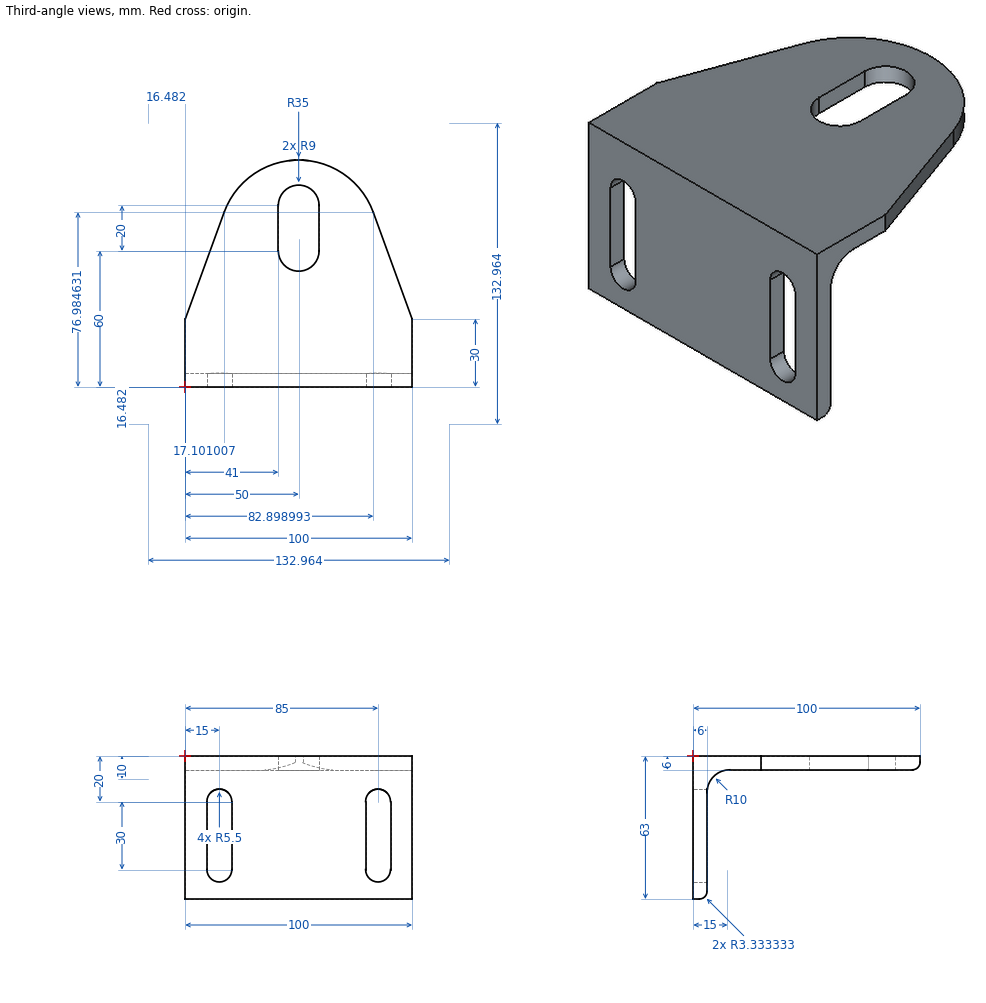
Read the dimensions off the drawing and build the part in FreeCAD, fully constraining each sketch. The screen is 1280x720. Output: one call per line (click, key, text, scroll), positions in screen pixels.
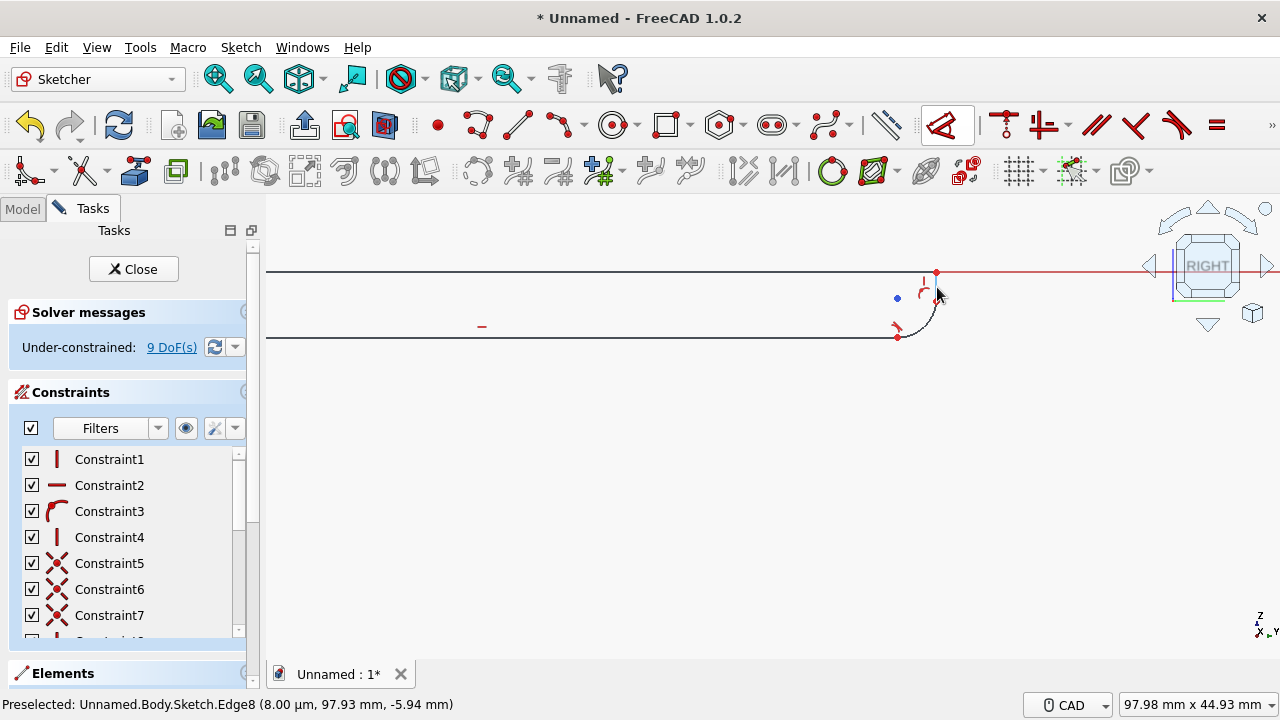
click(936, 287)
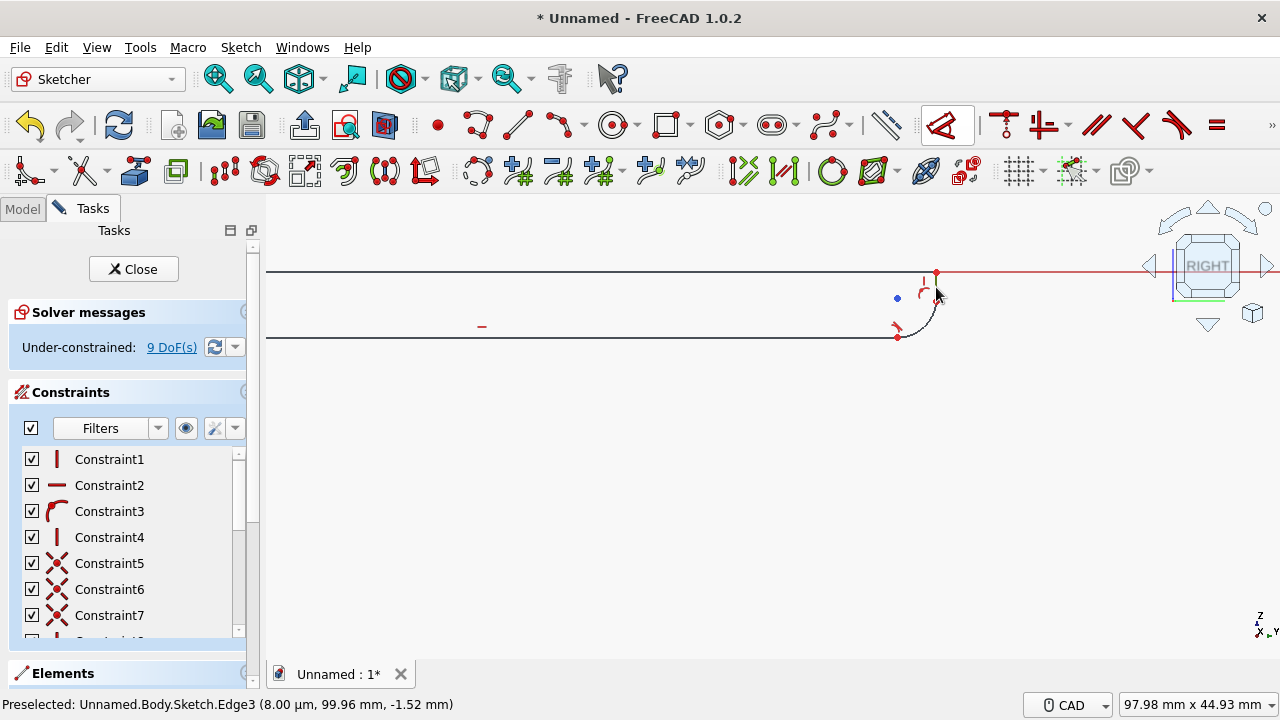
click(914, 334)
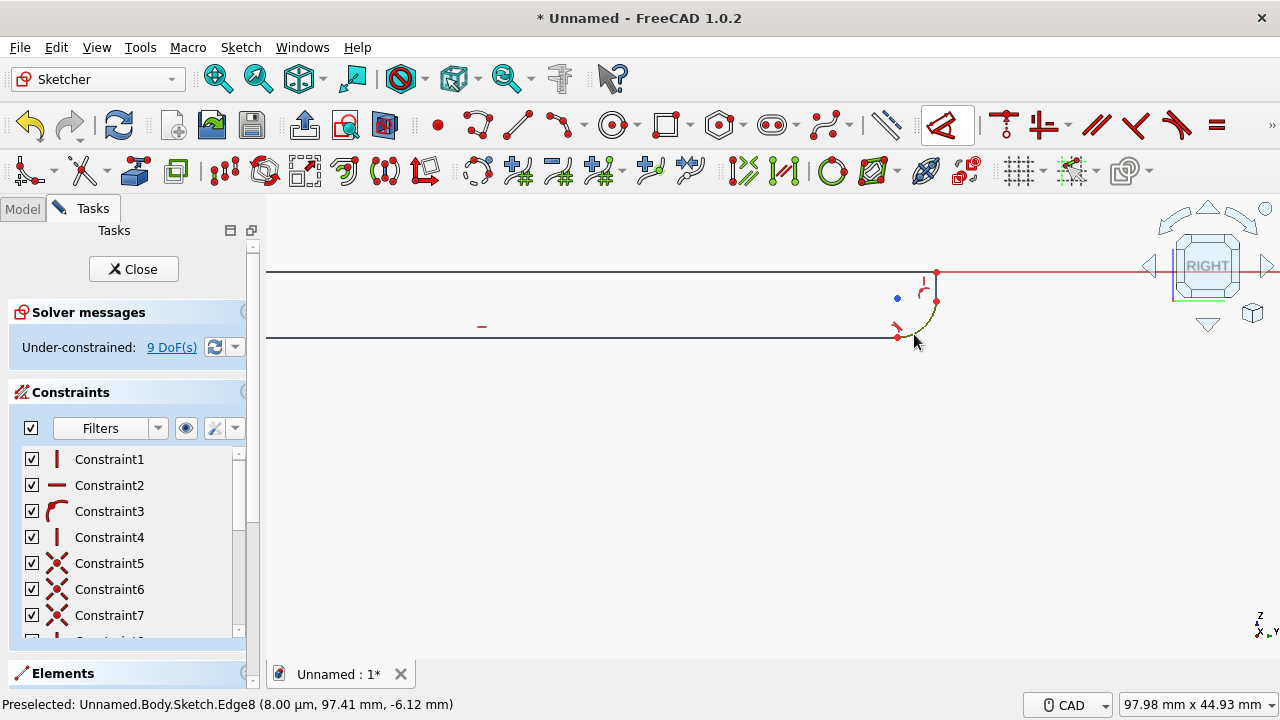
click(1178, 126)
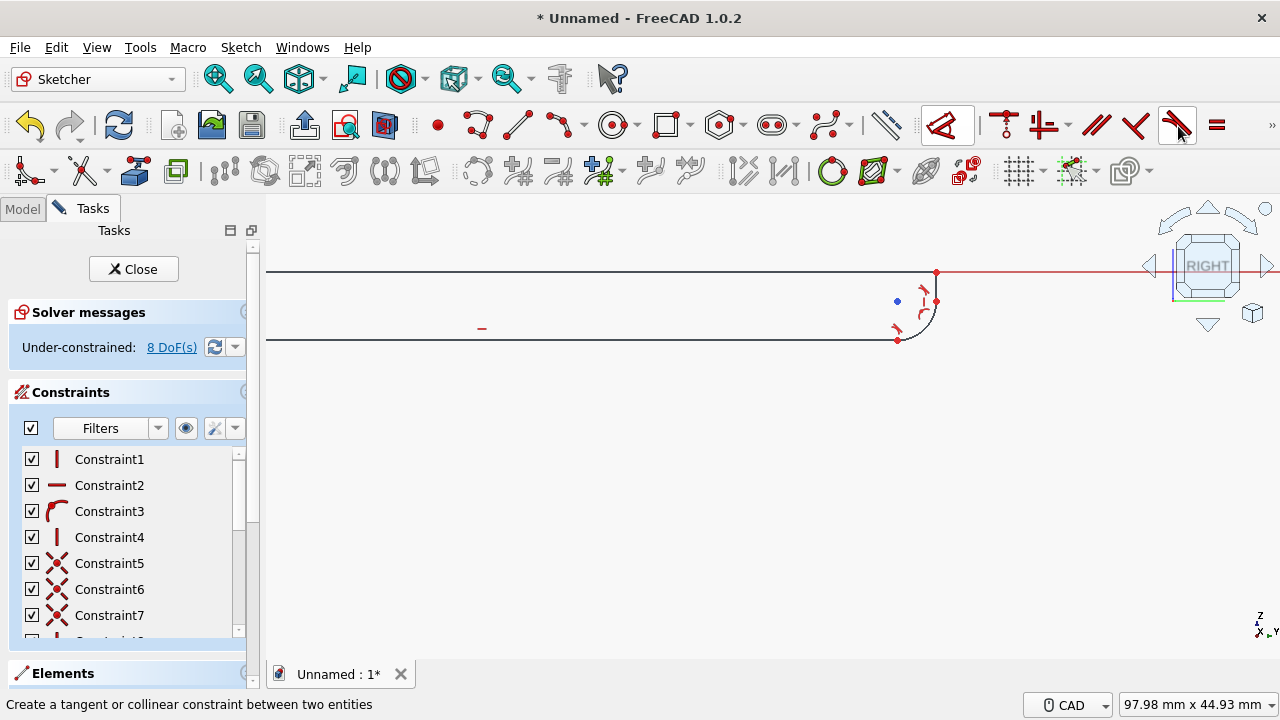
scroll(937, 286, down, 4)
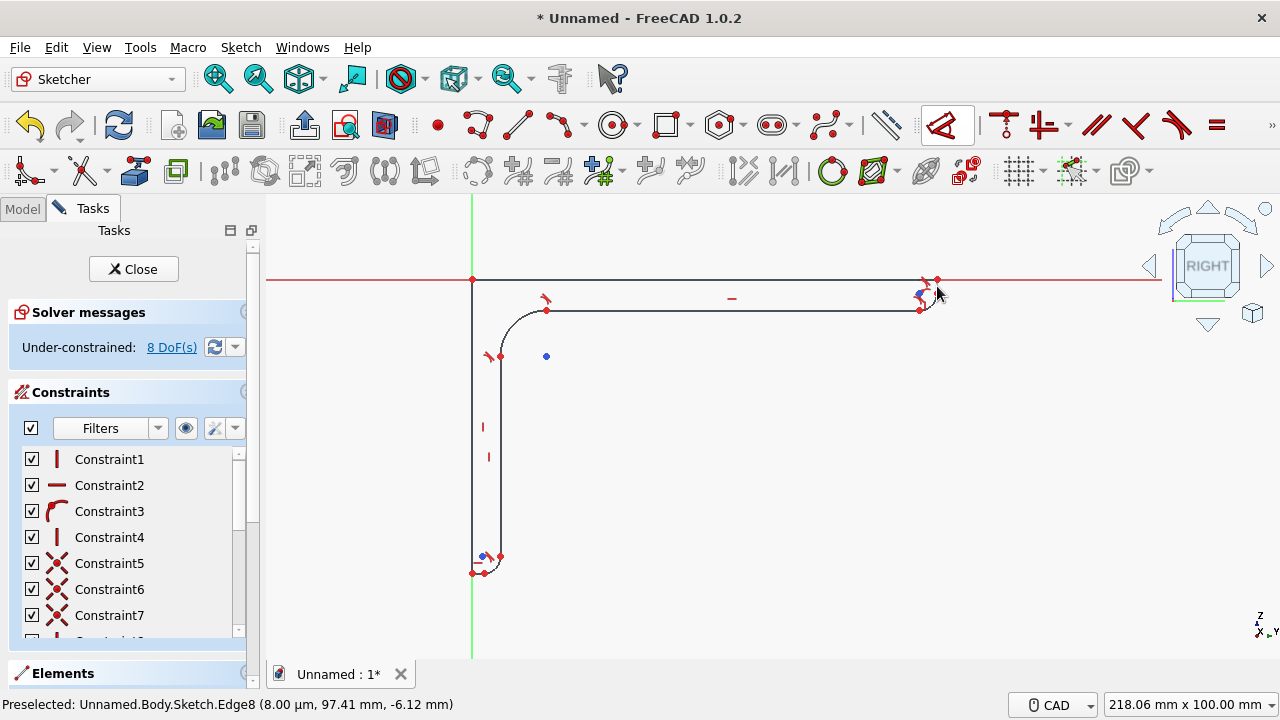
scroll(477, 574, up, 5)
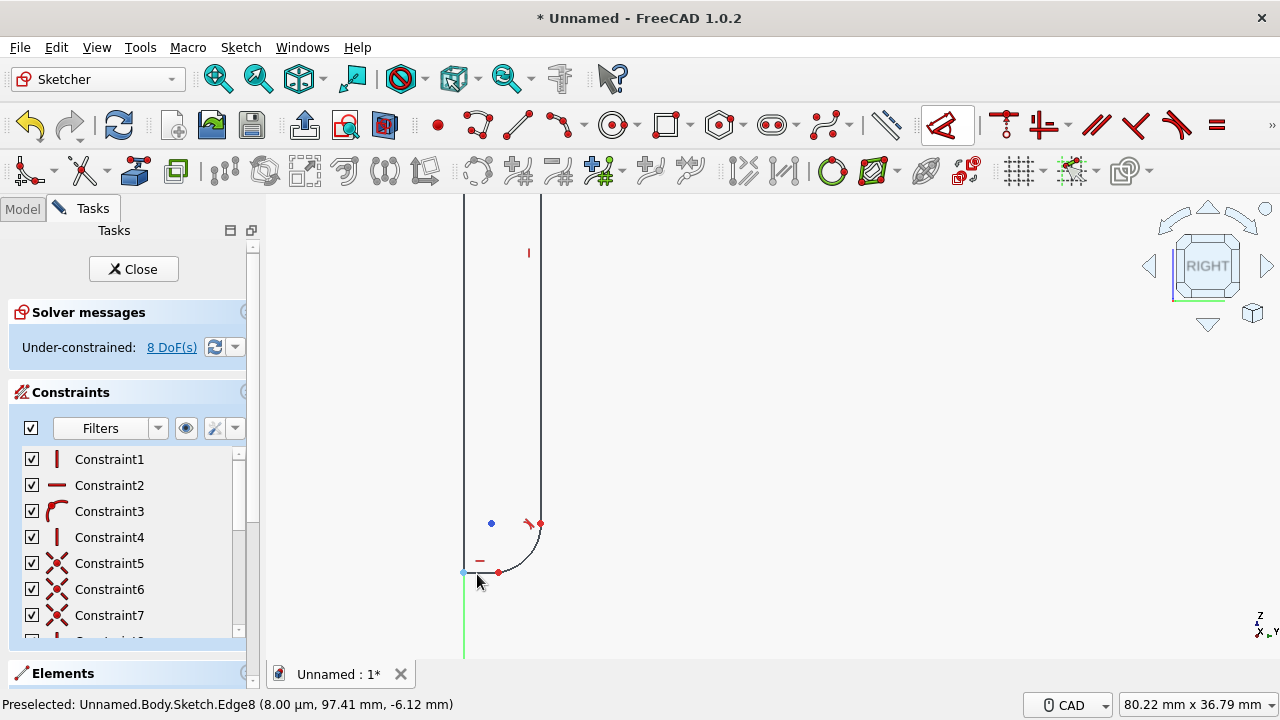
click(478, 573)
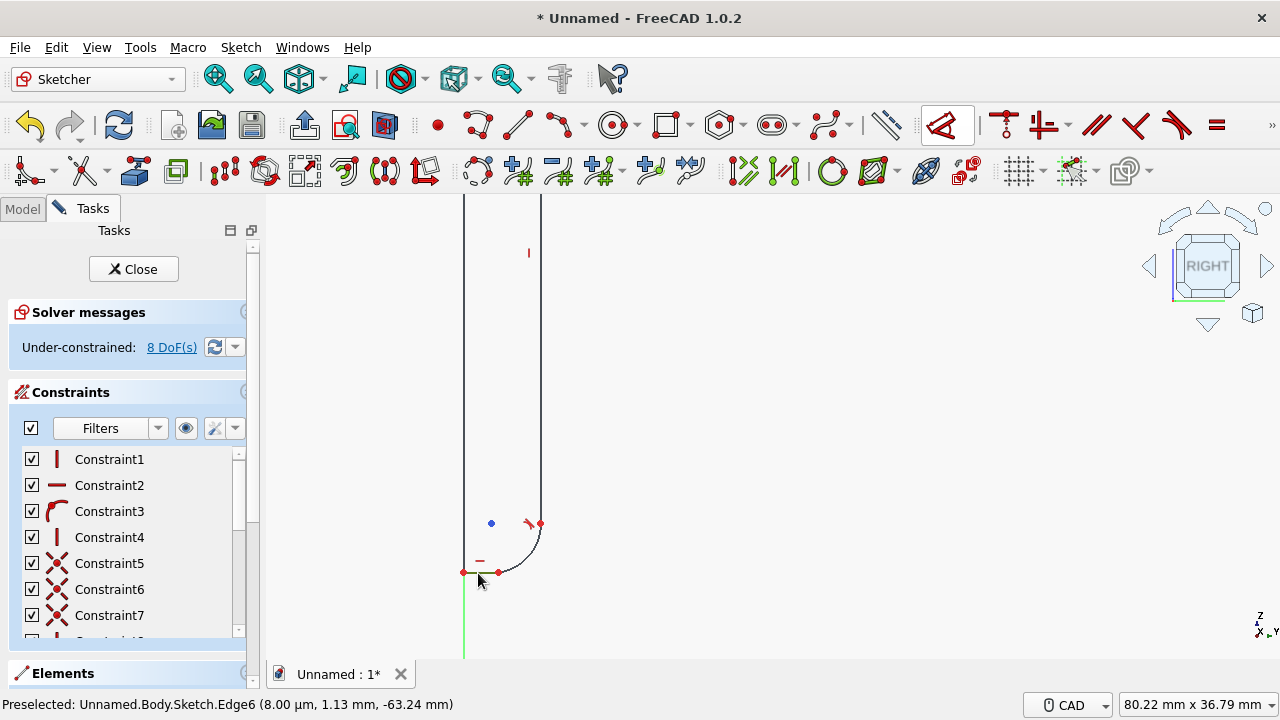
click(518, 565)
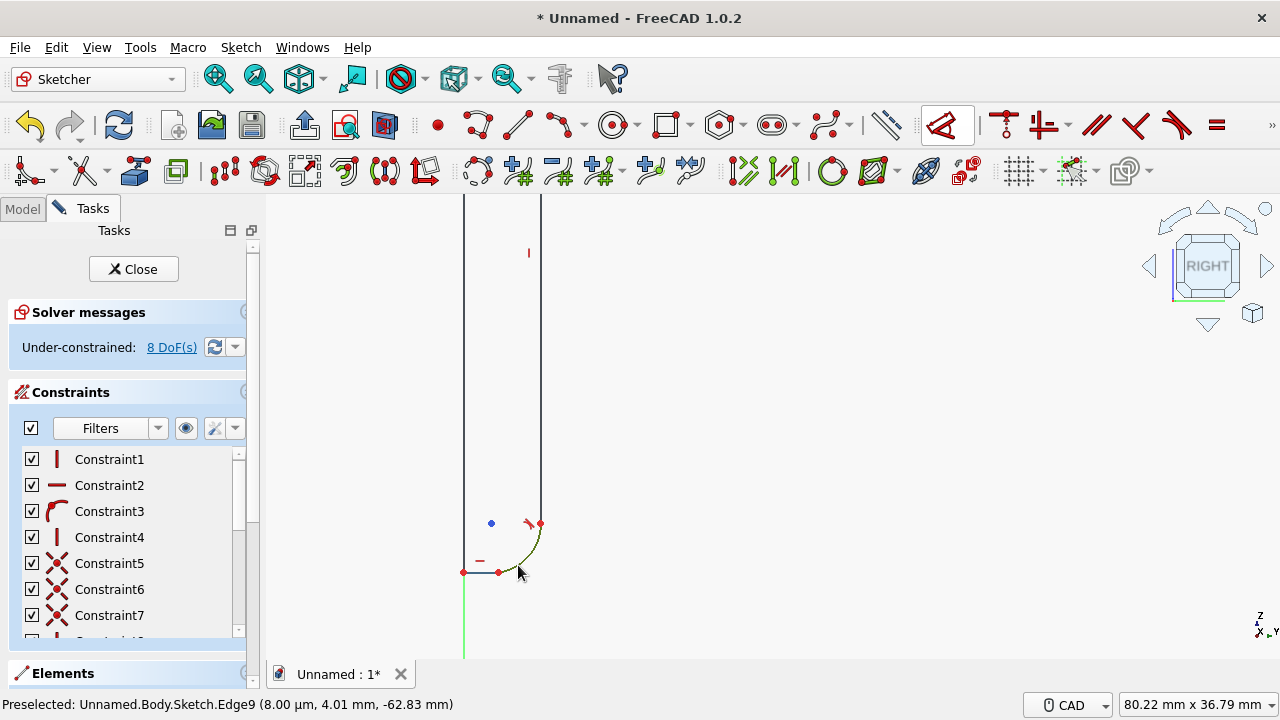
click(1178, 126)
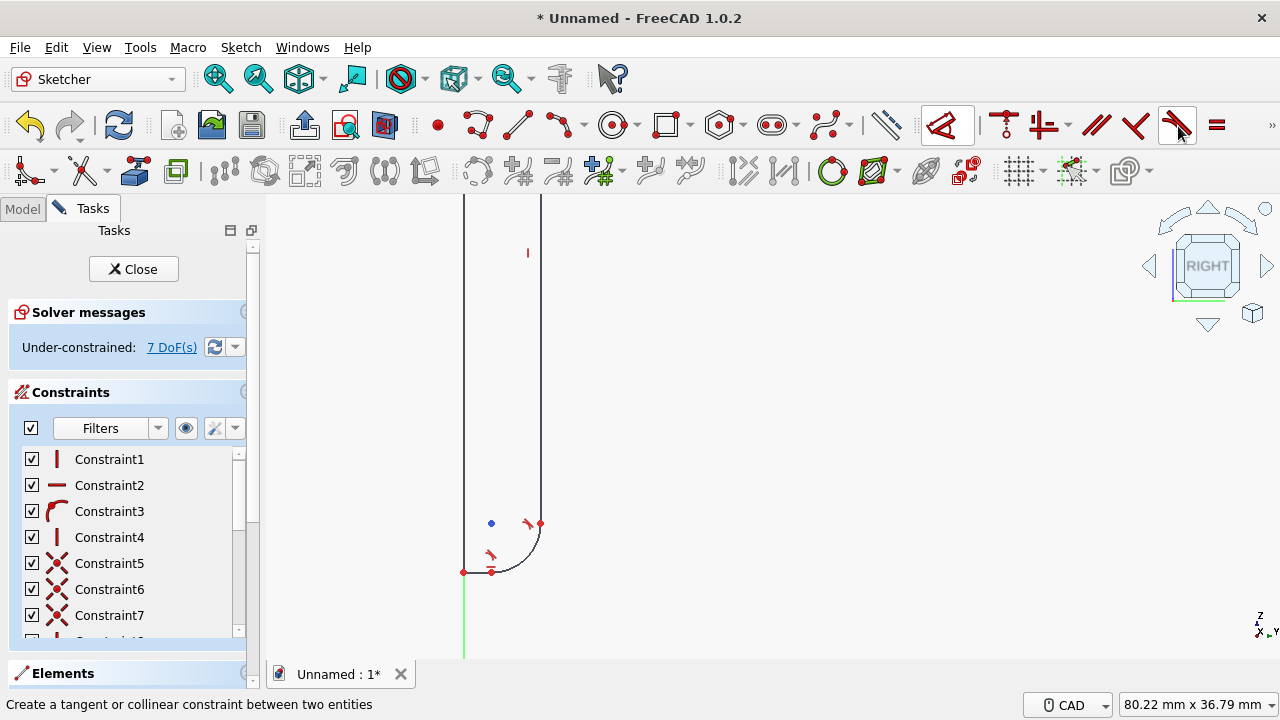
scroll(477, 575, down, 5)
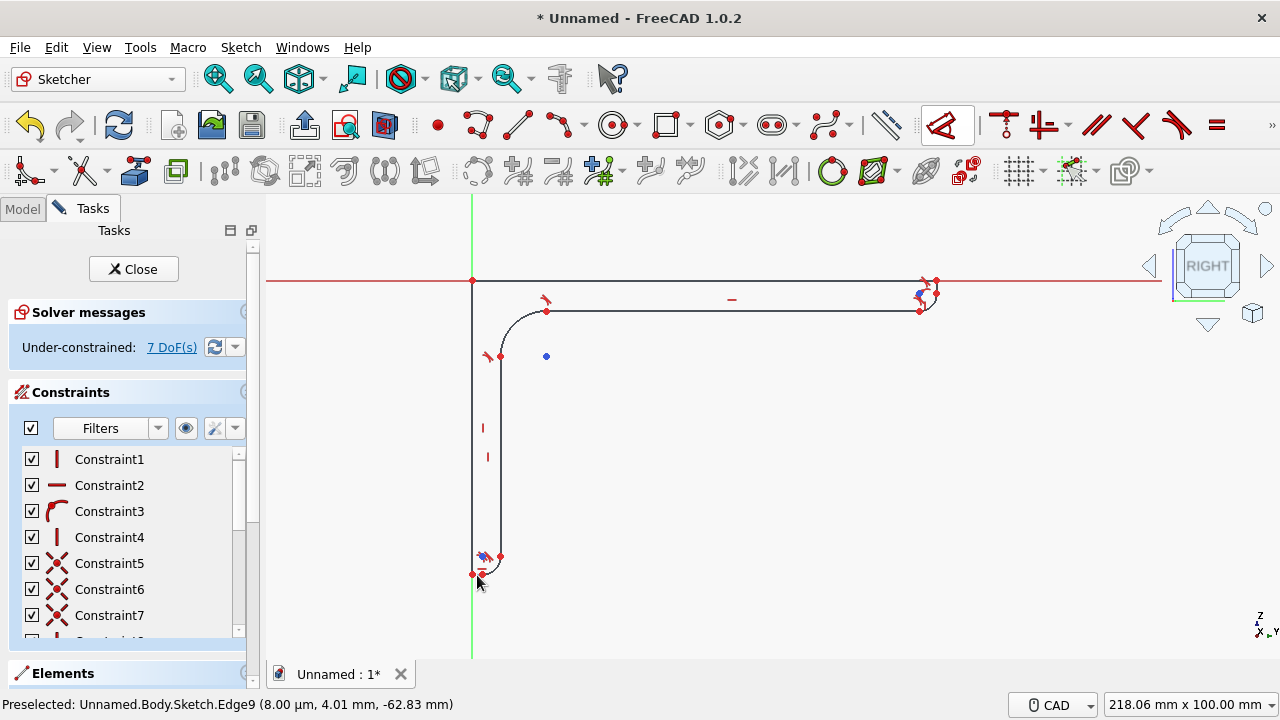
scroll(927, 309, up, 3)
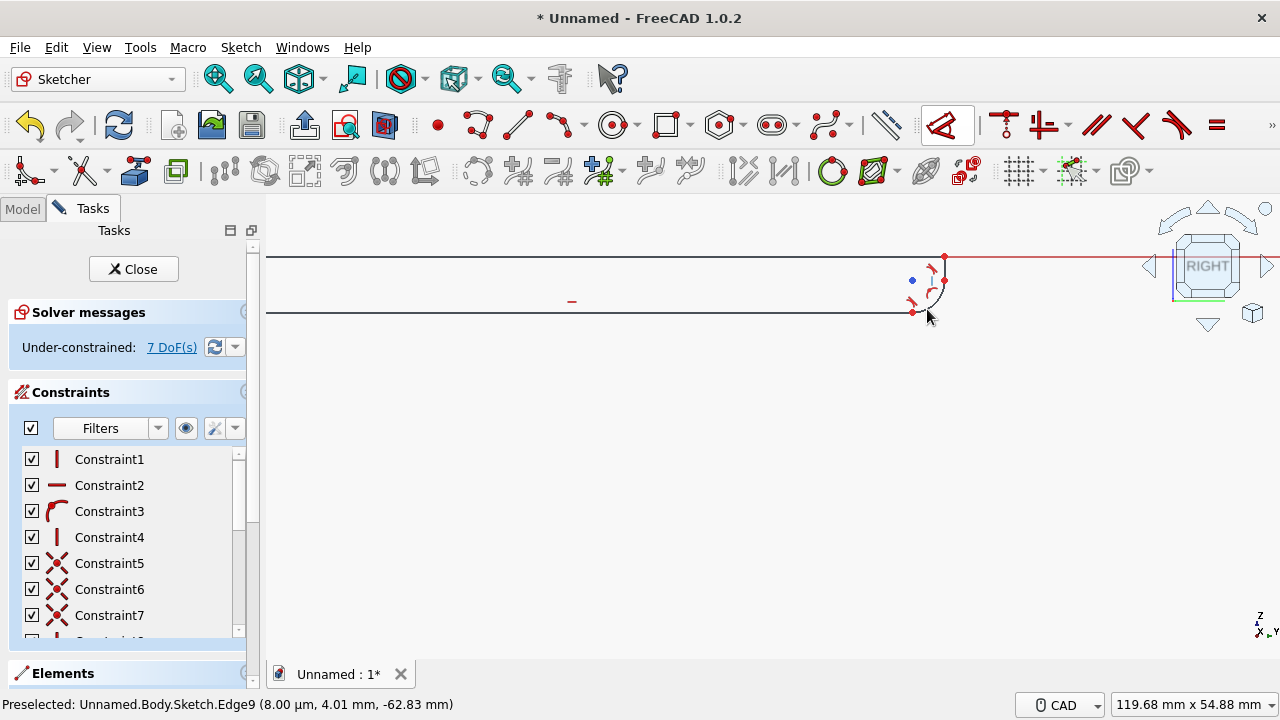
click(927, 309)